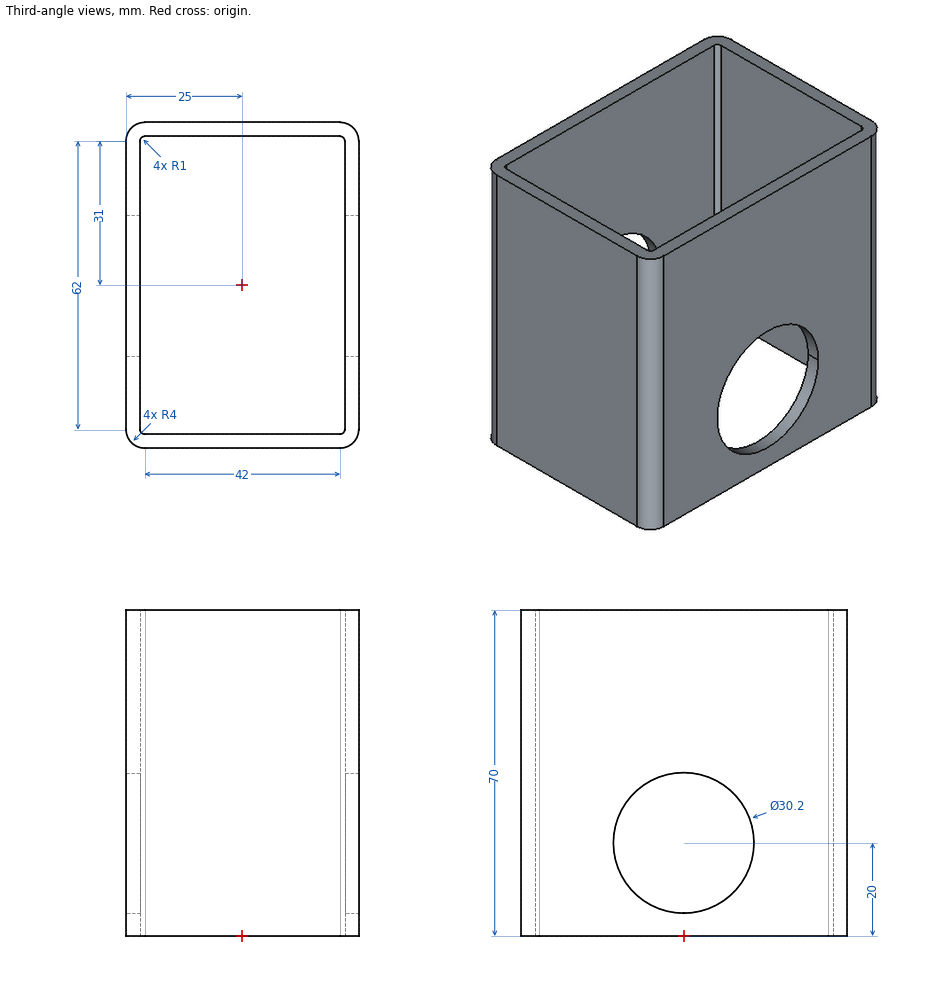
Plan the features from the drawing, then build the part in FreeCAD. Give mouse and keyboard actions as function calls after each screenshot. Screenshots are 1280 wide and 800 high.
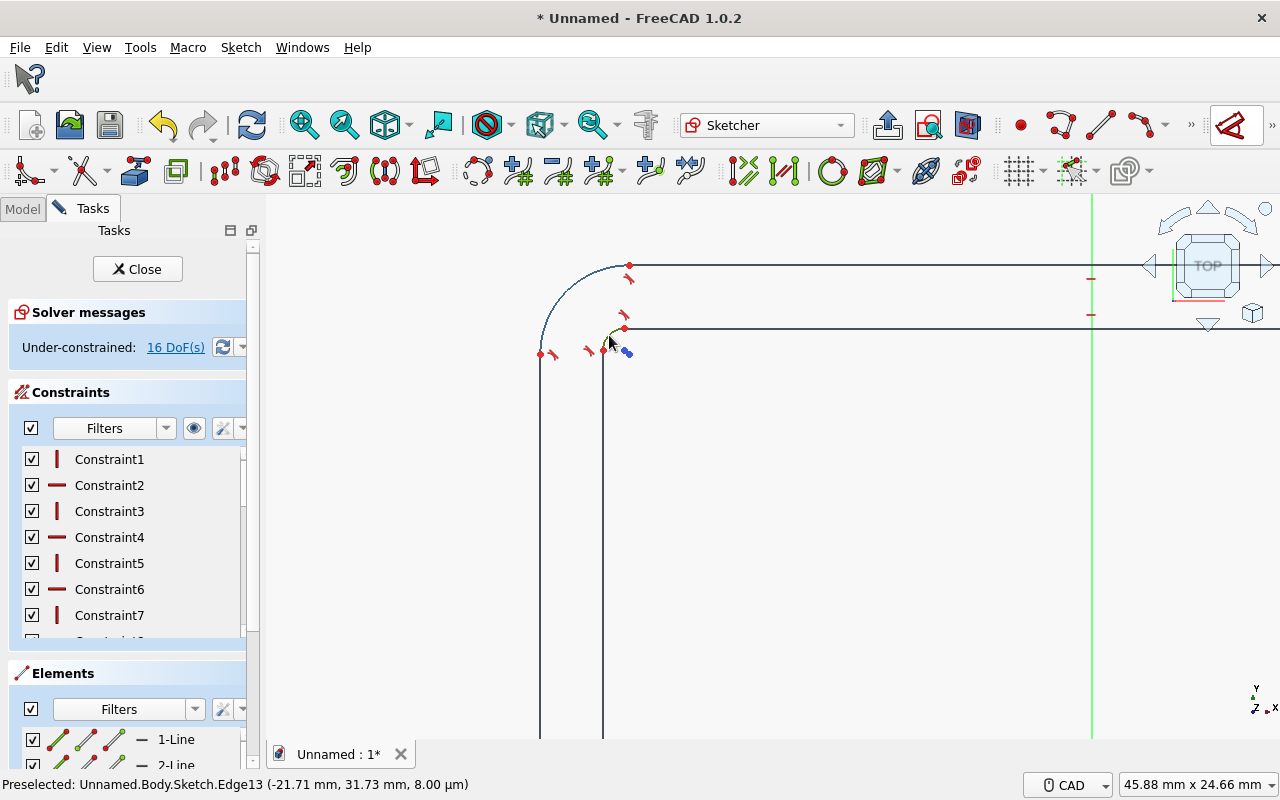
key(c)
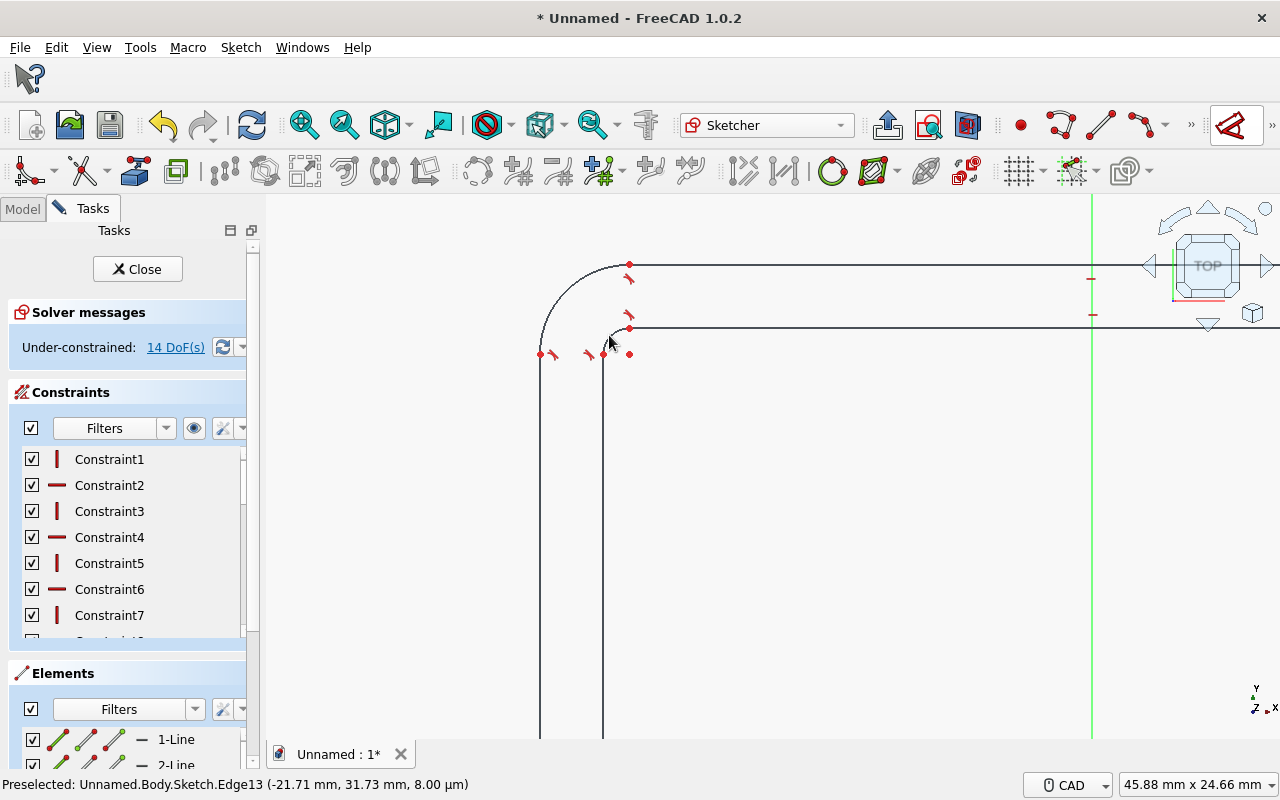
scroll(607, 323, down, 8)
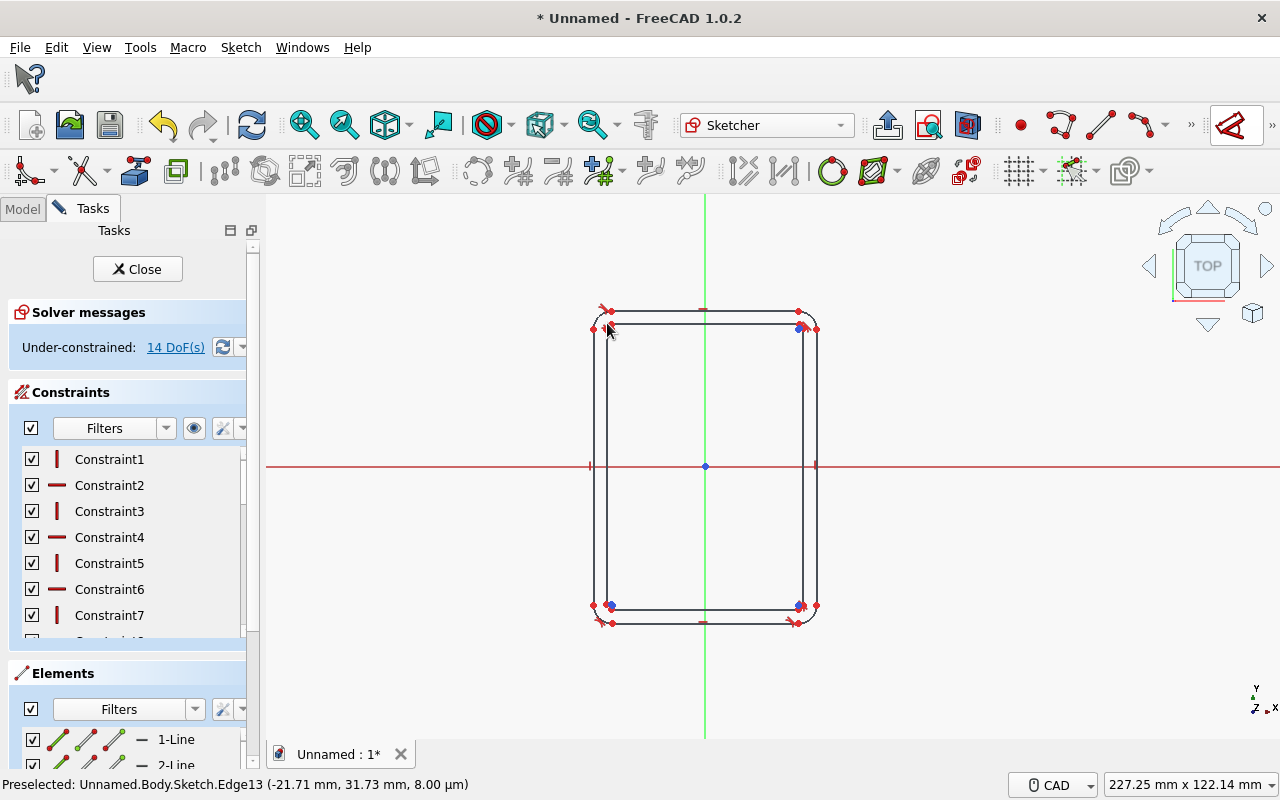
scroll(815, 321, up, 3)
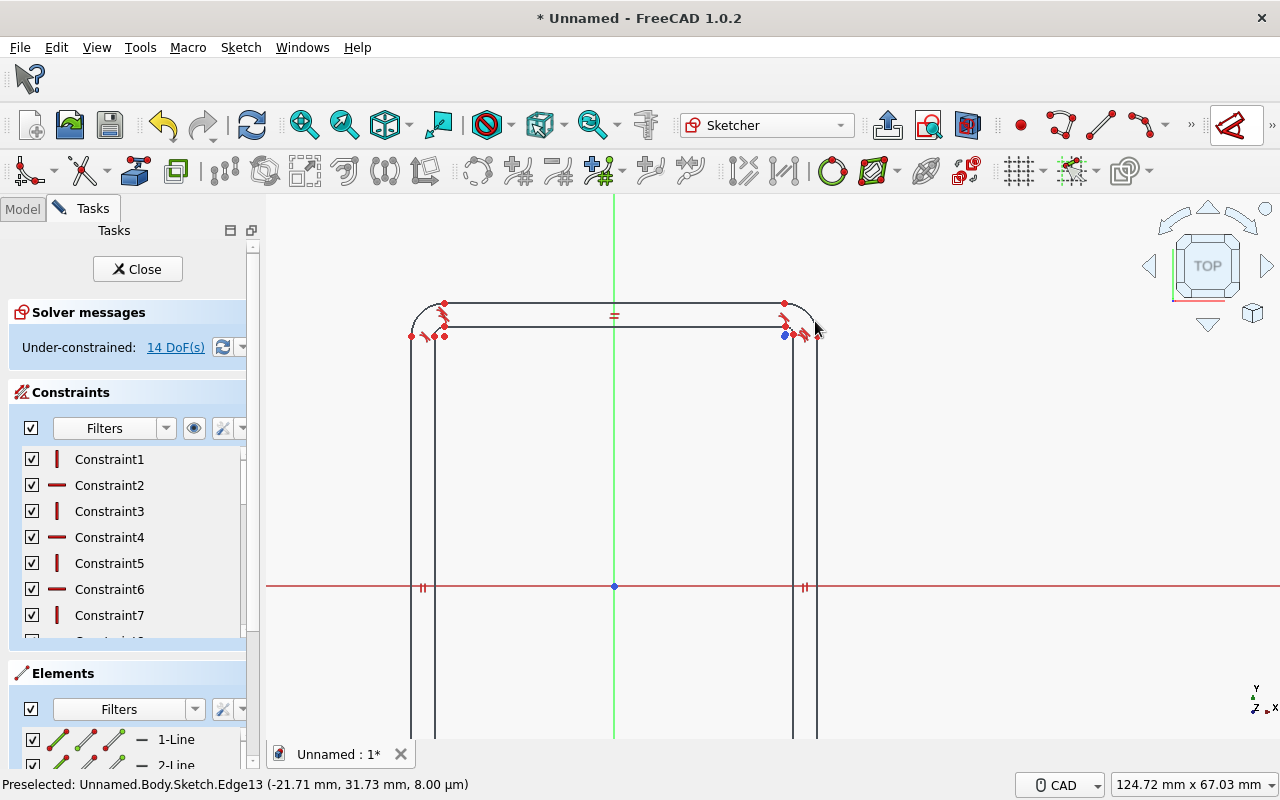
click(814, 321)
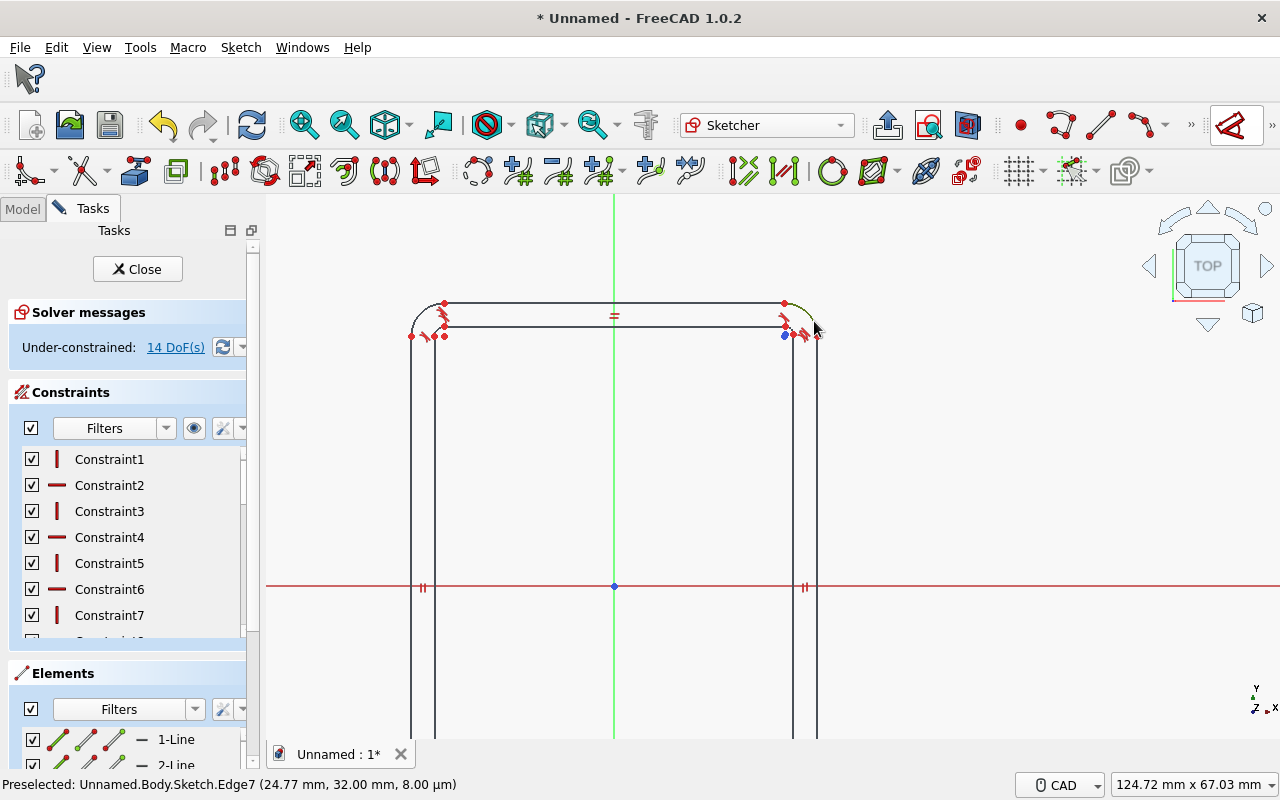
scroll(791, 329, up, 5)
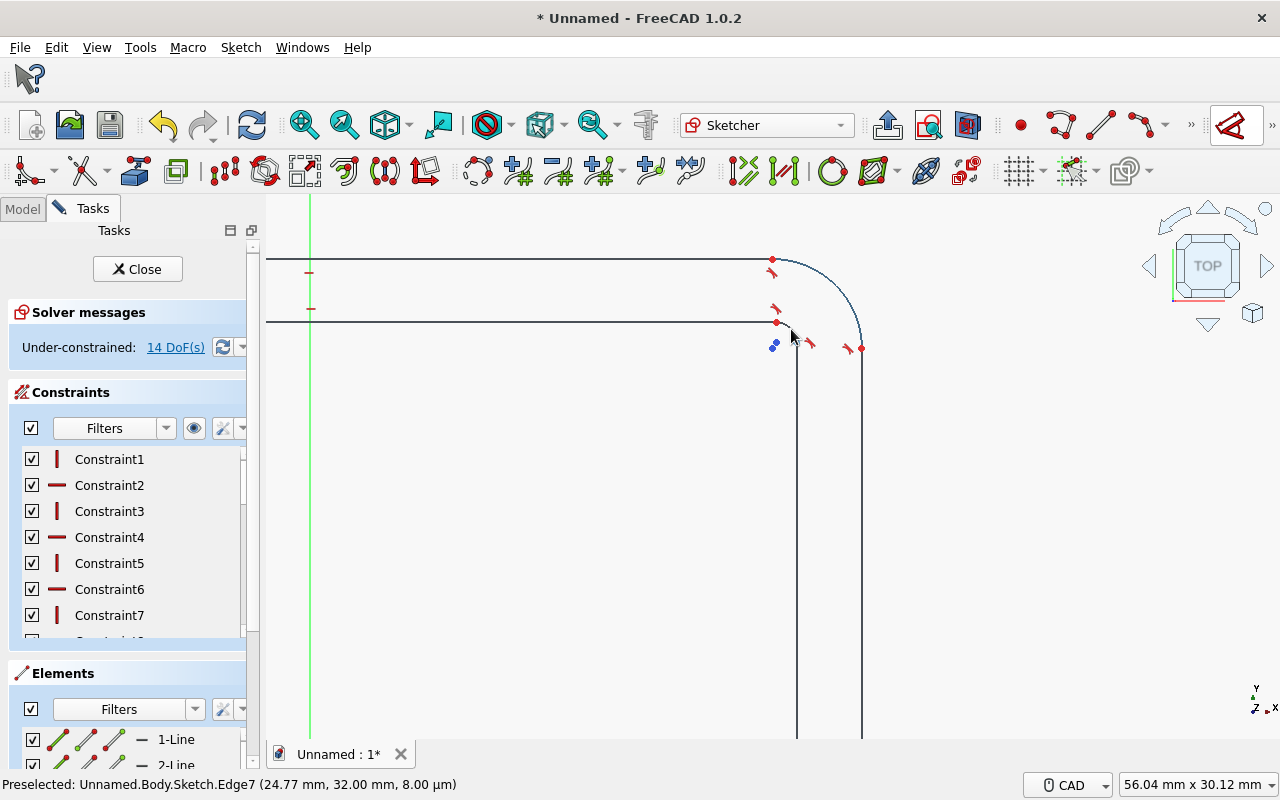
click(791, 328)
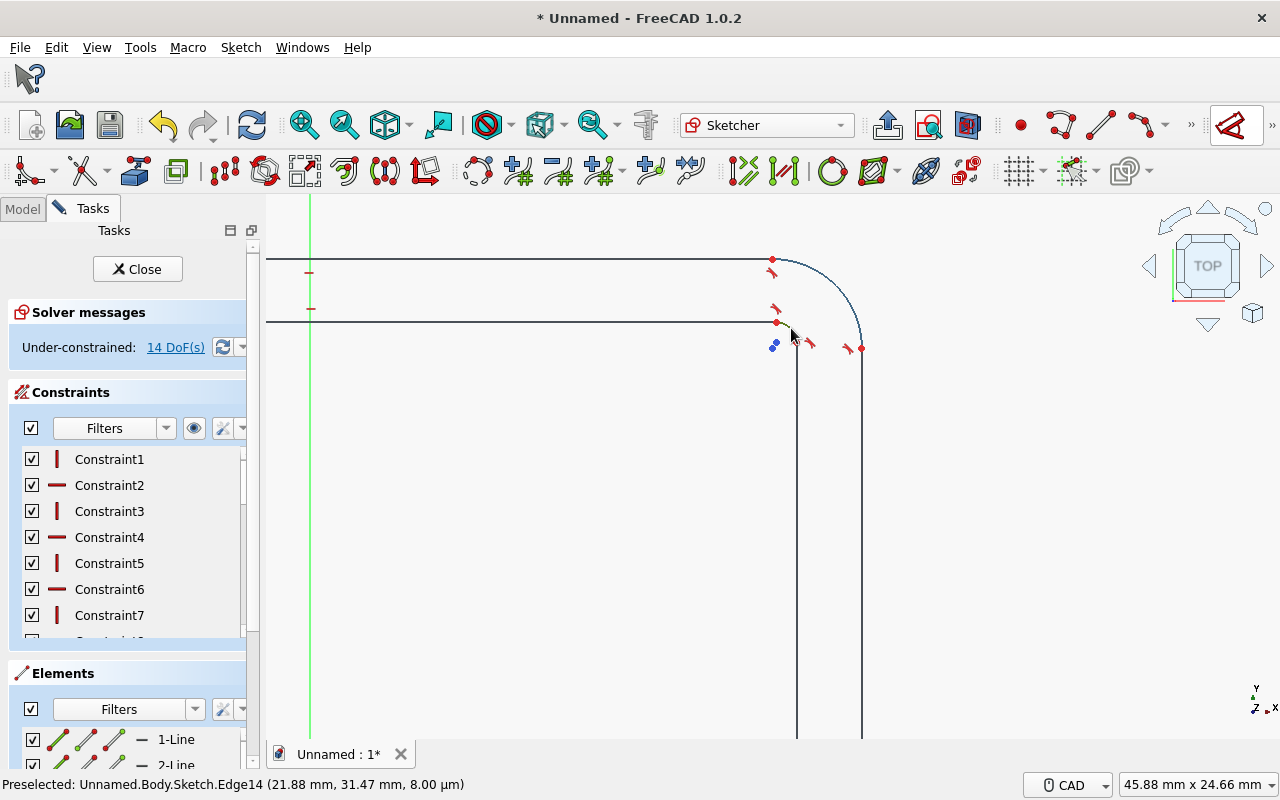
key(c)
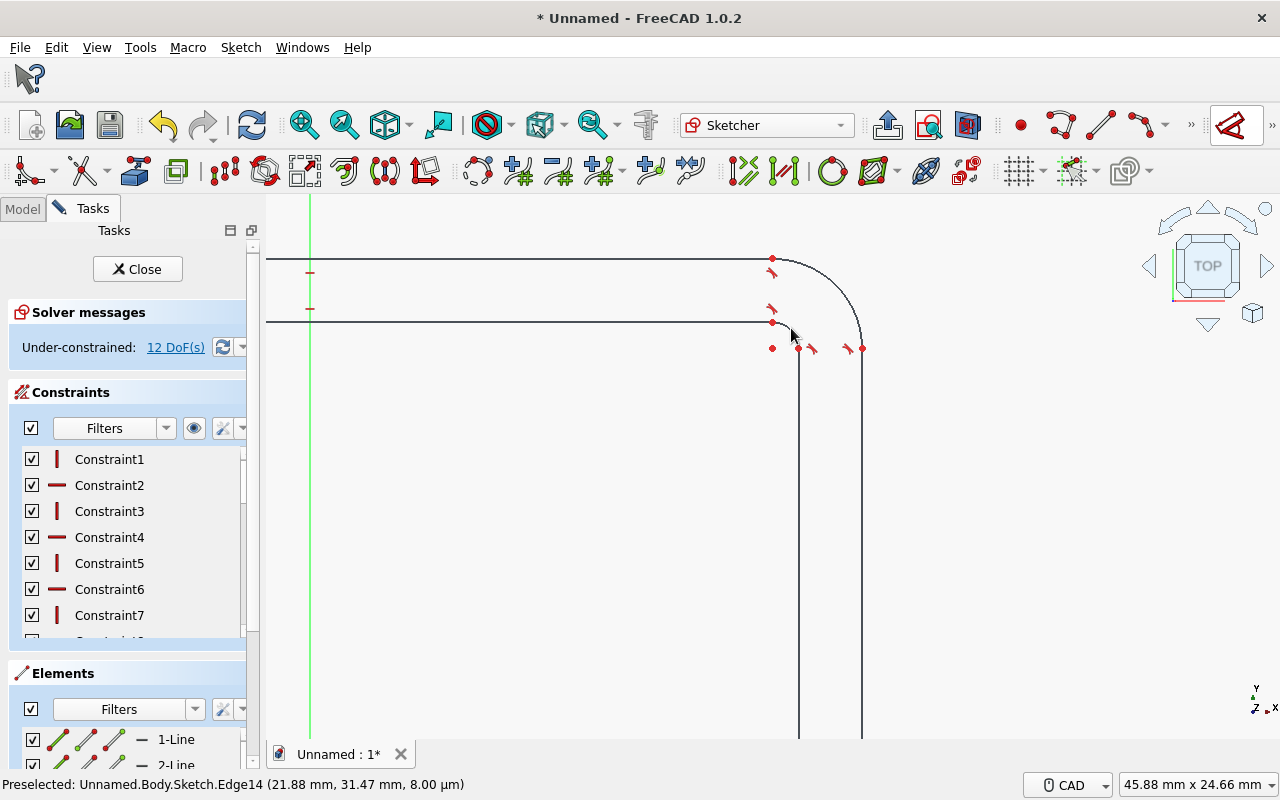
scroll(804, 324, down, 8)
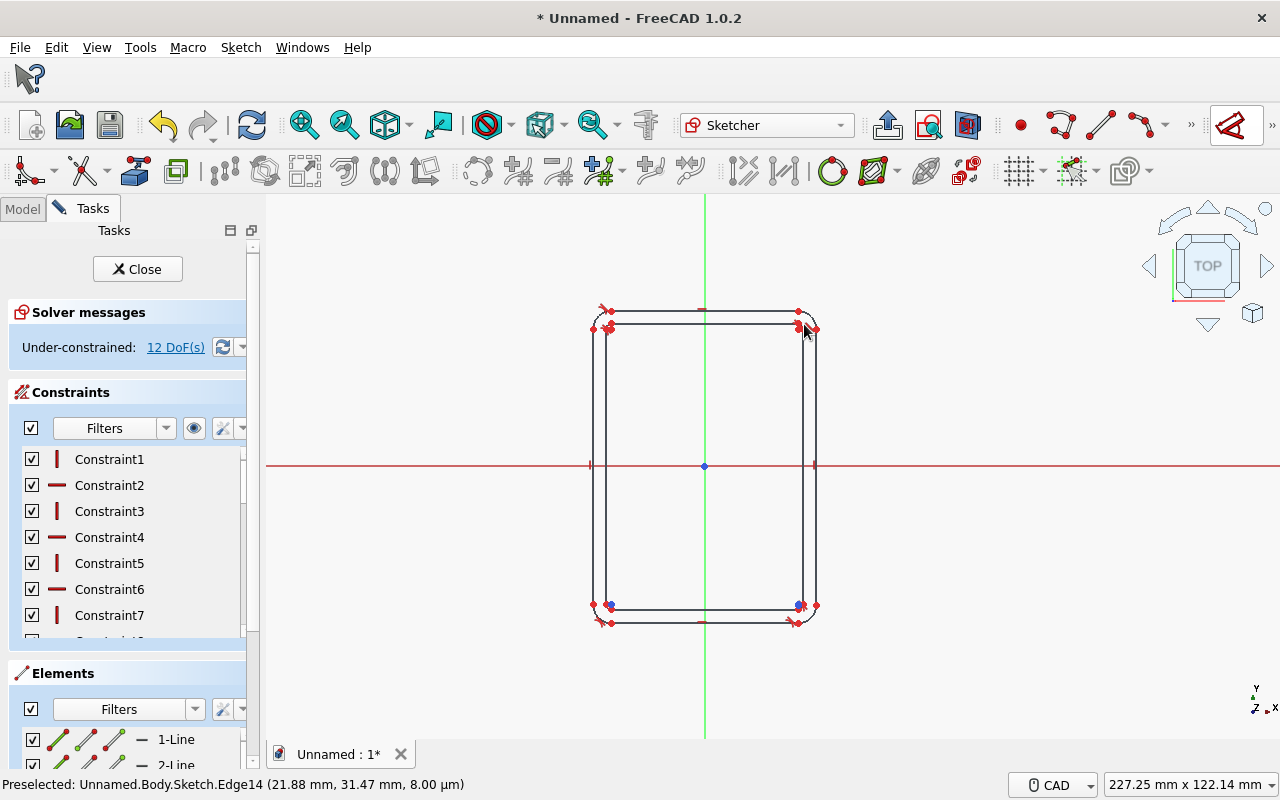
scroll(806, 621, up, 3)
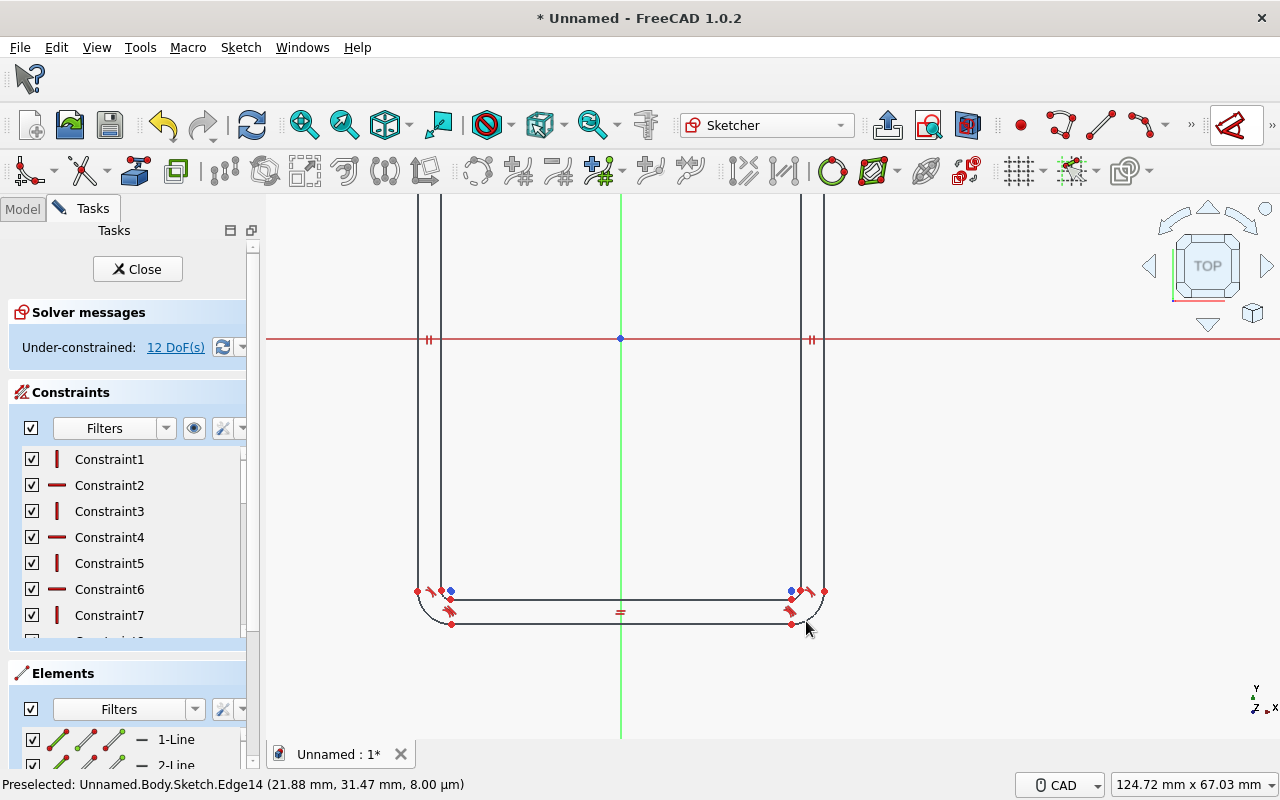
click(806, 621)